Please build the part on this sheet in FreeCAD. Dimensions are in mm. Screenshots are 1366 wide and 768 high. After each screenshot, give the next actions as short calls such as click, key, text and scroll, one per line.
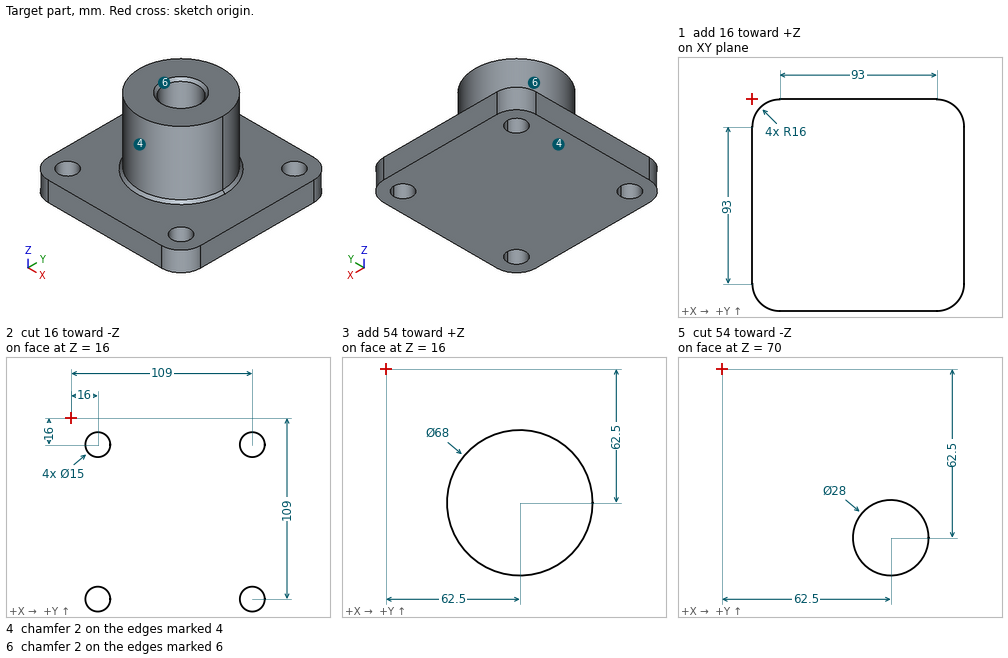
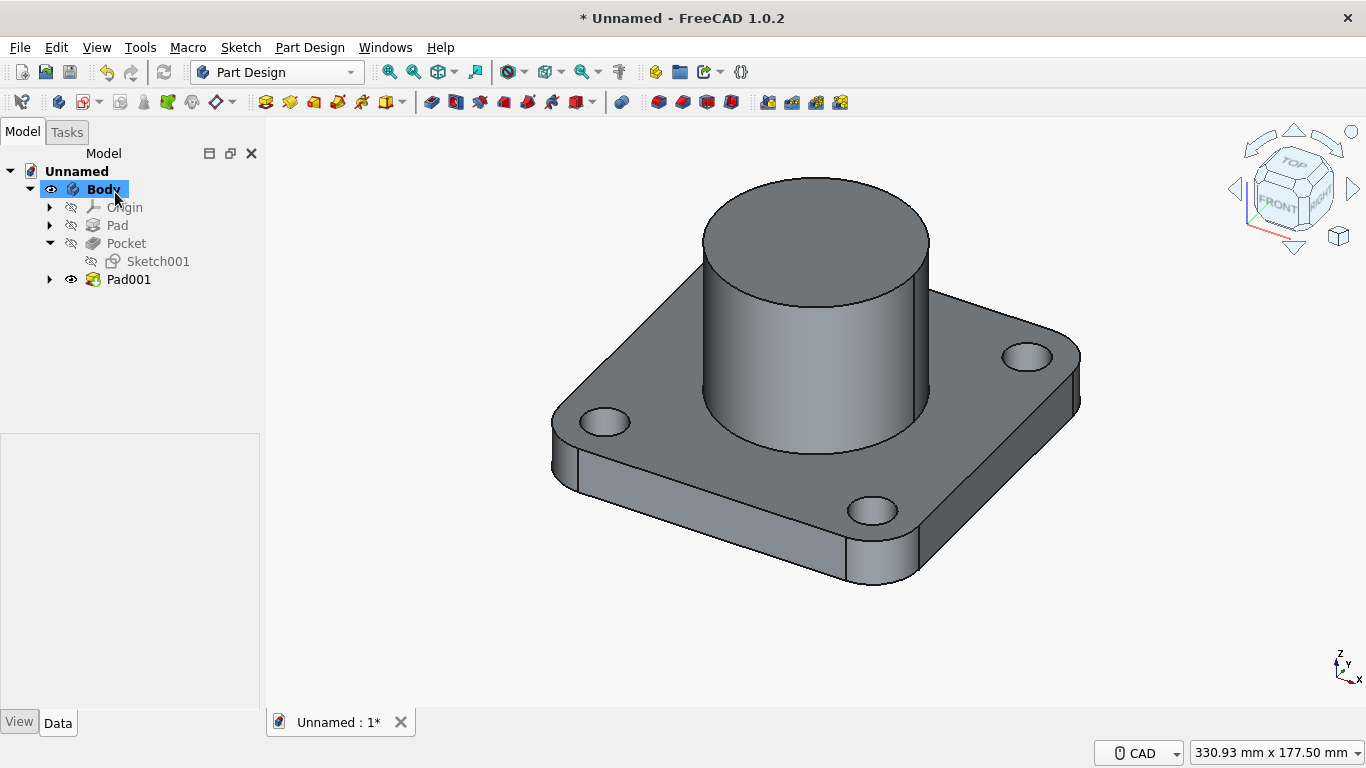
key(v)
key(f)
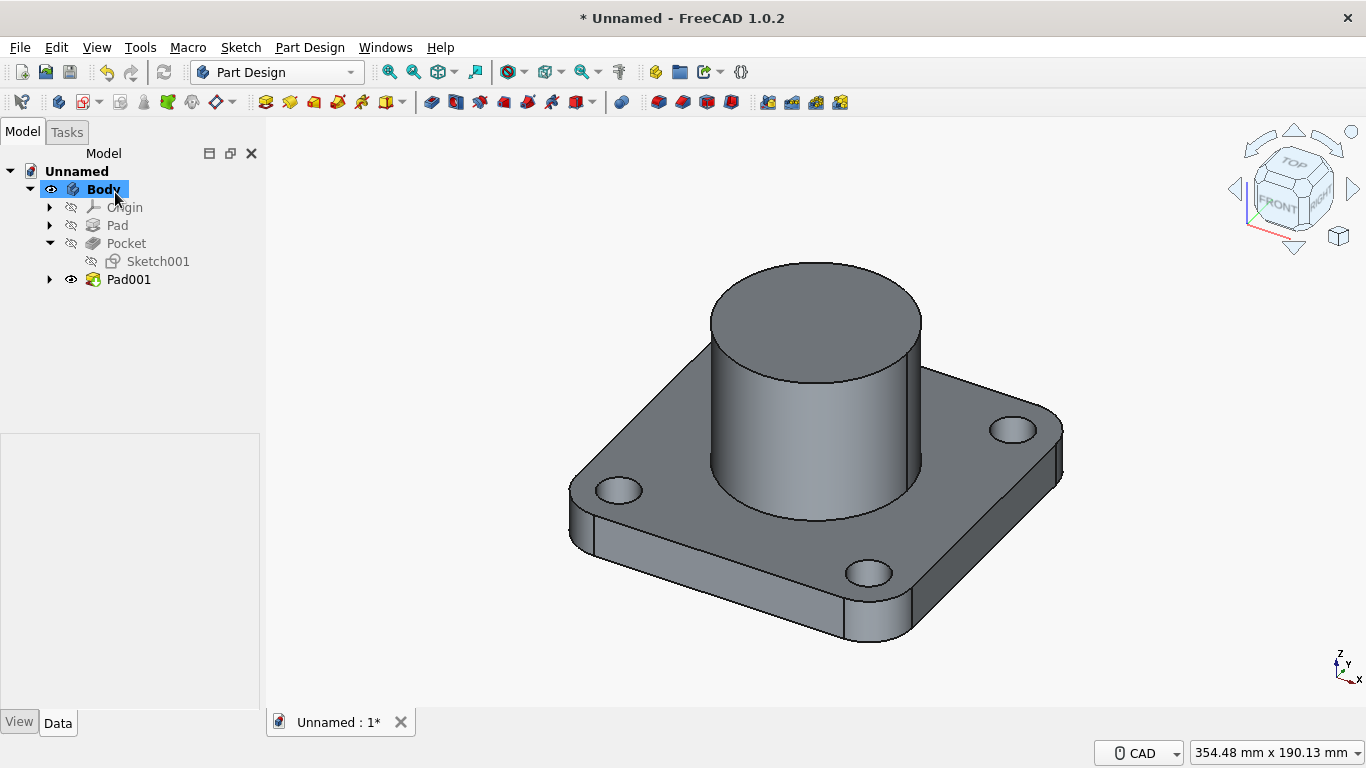
key(0)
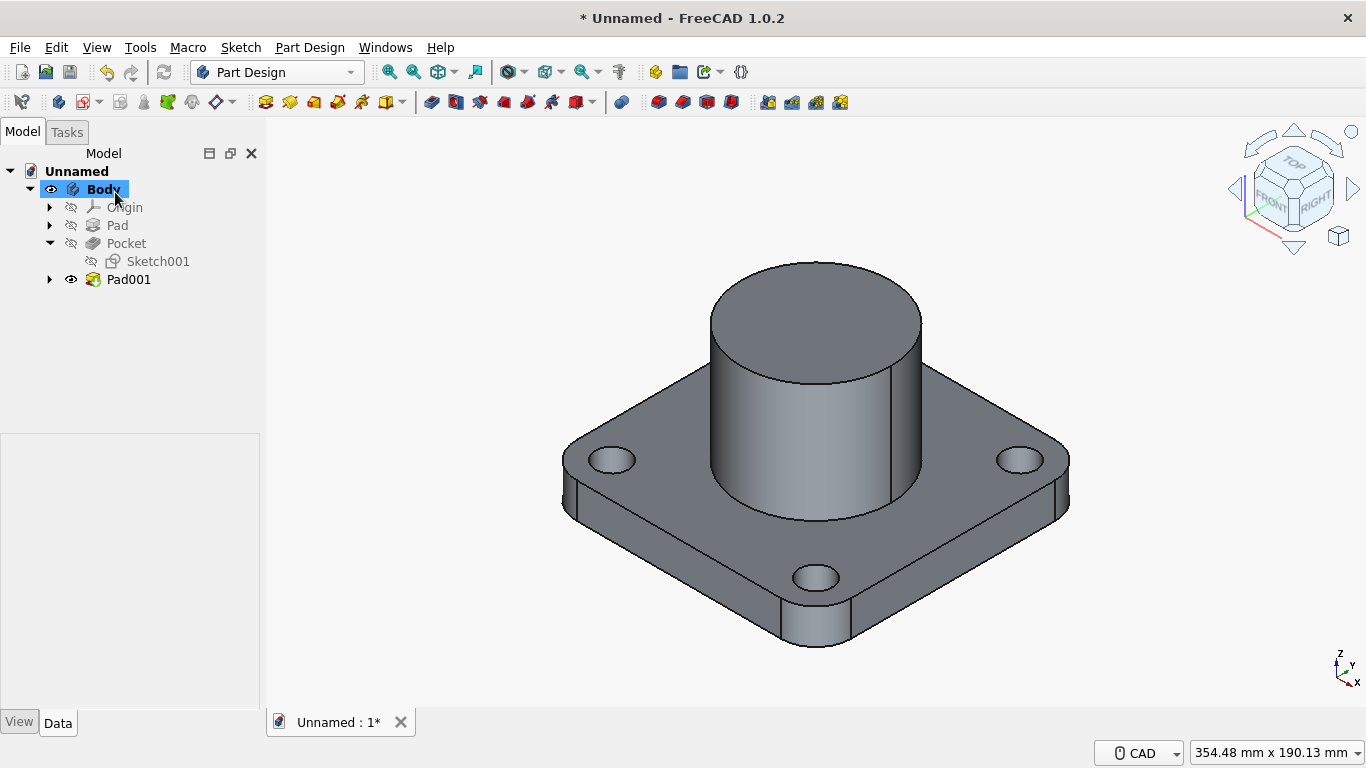
key(2)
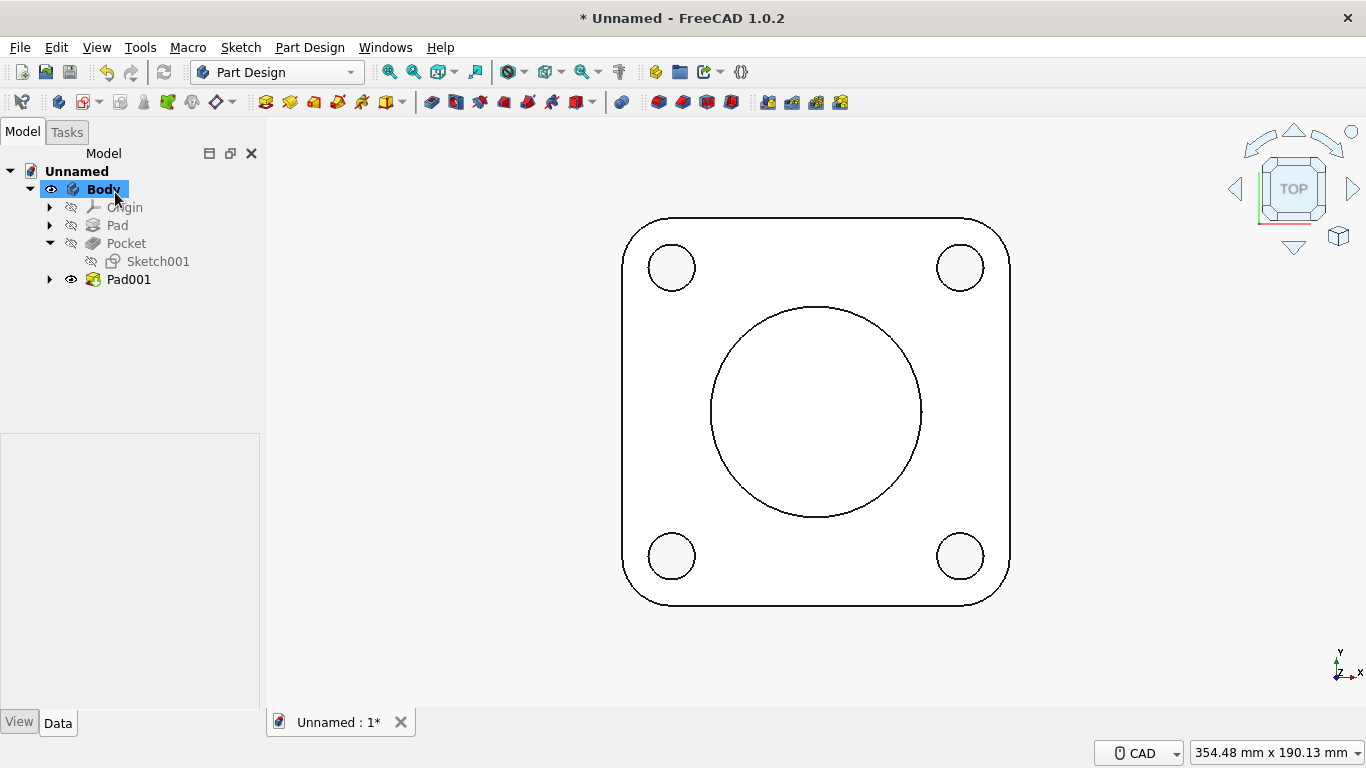
key(1)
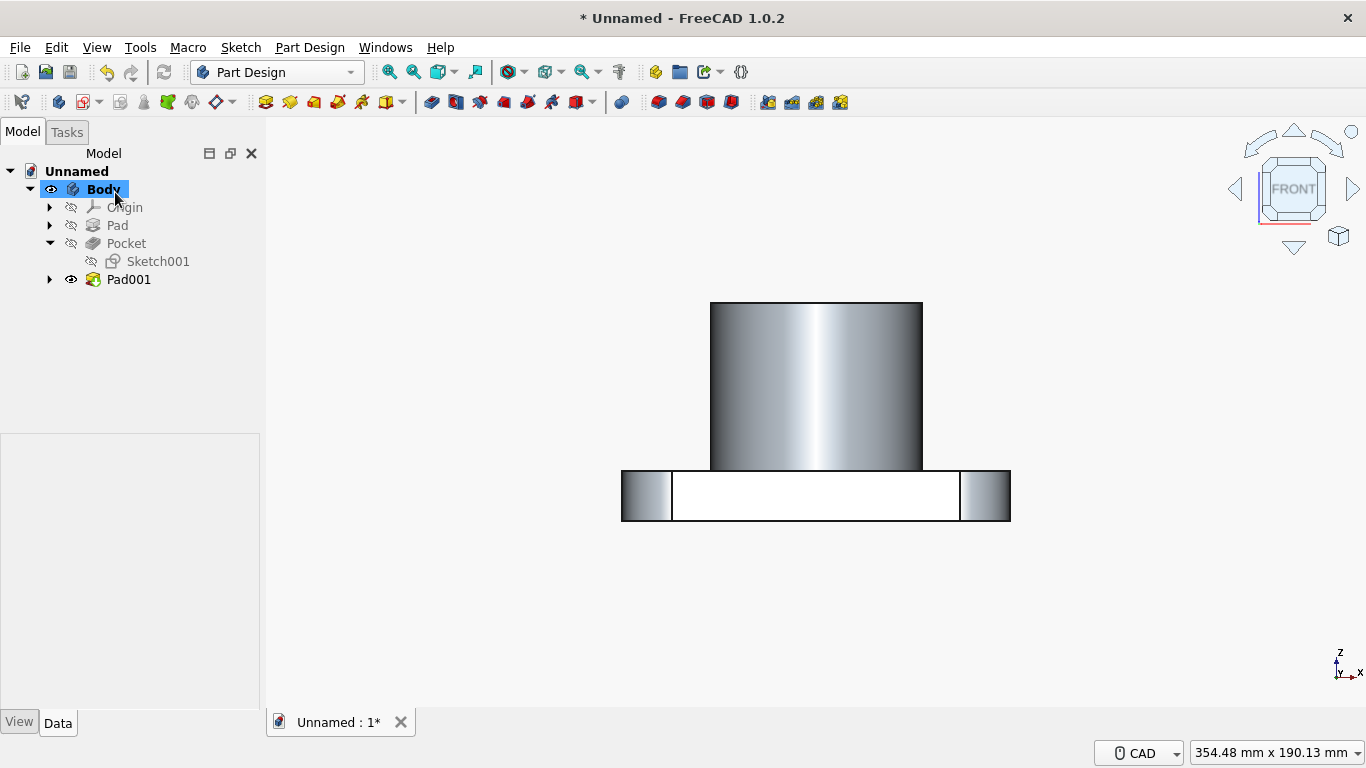
key(v)
key(f)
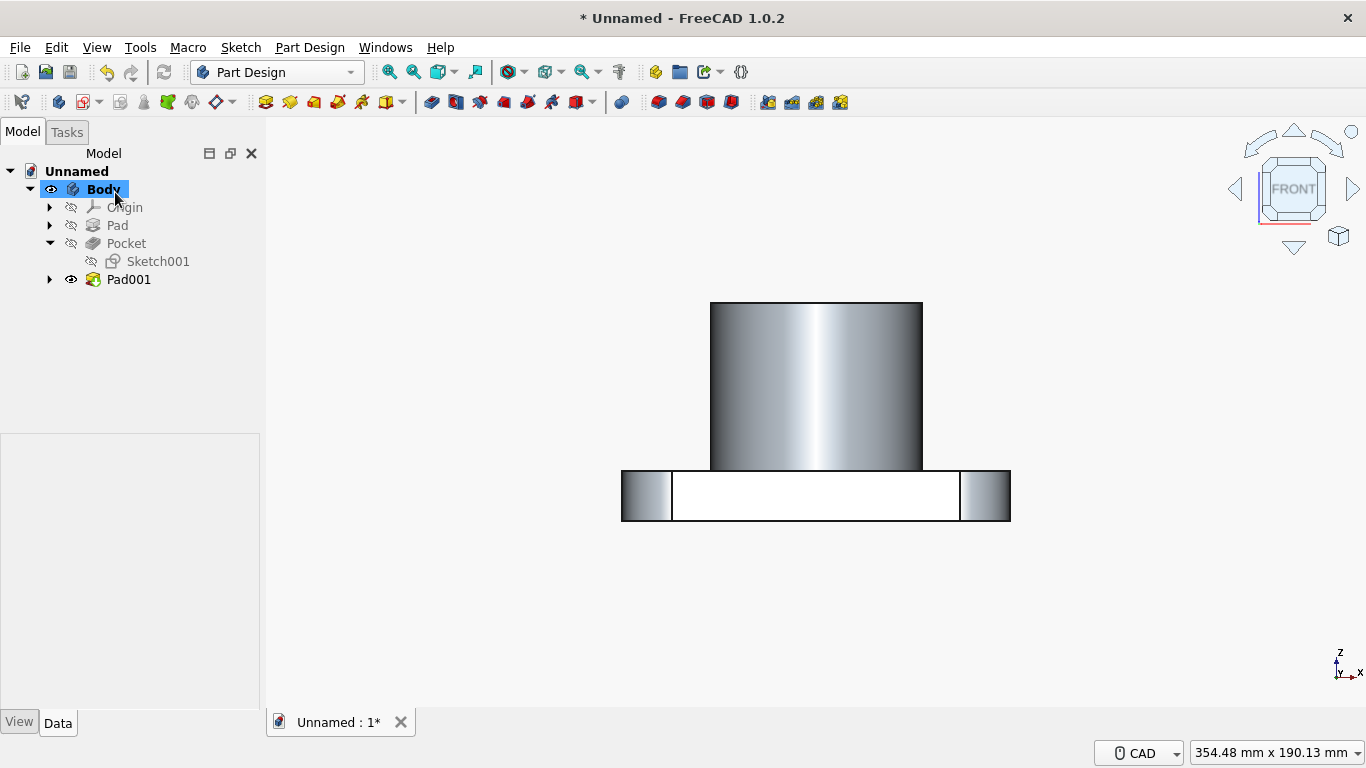
key(3)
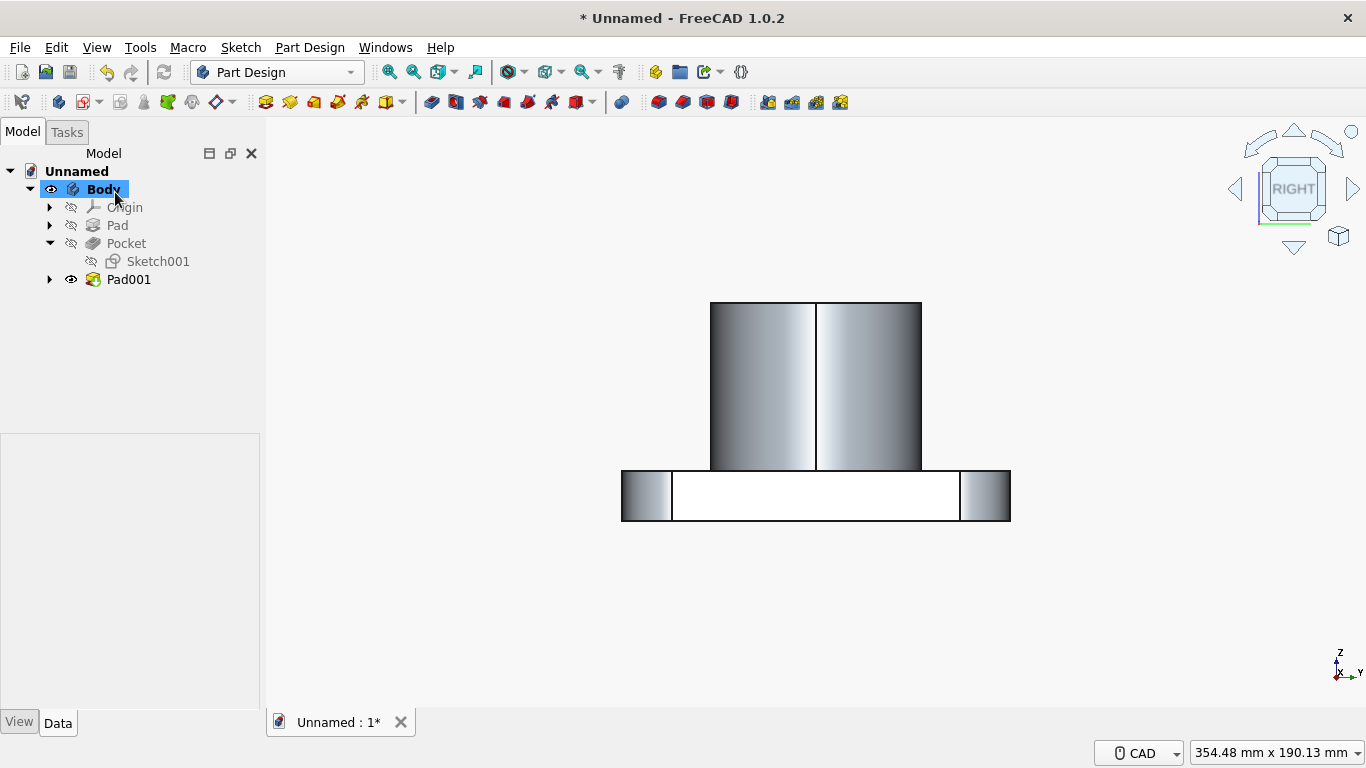
key(v)
key(f)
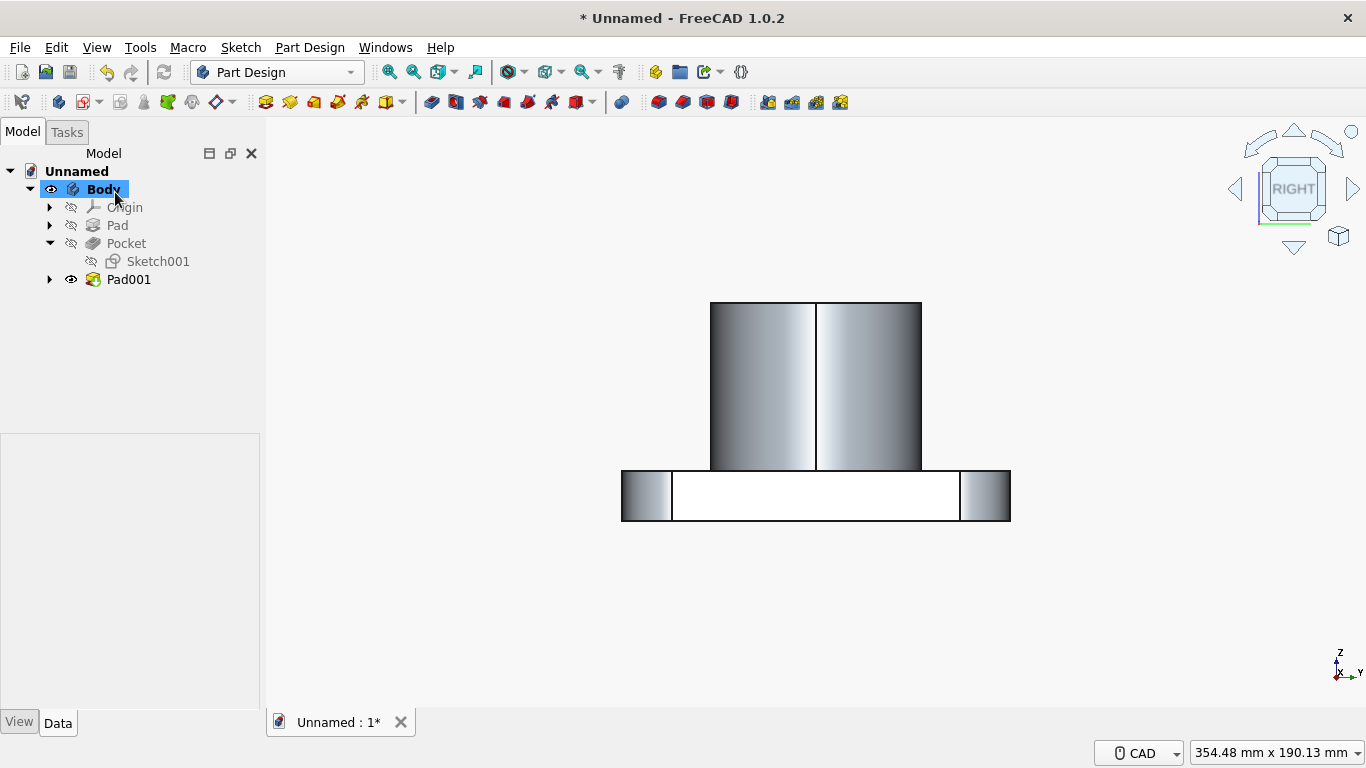
key(5)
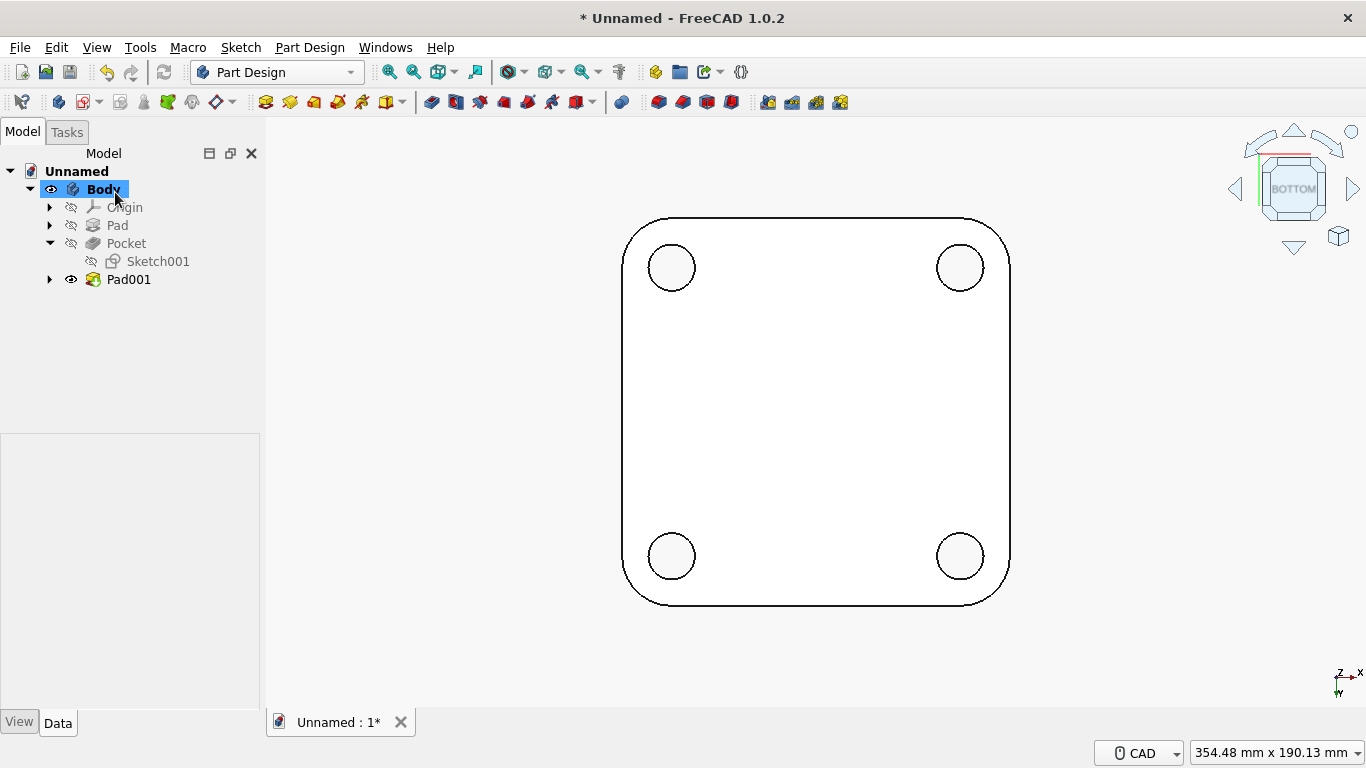
key(4)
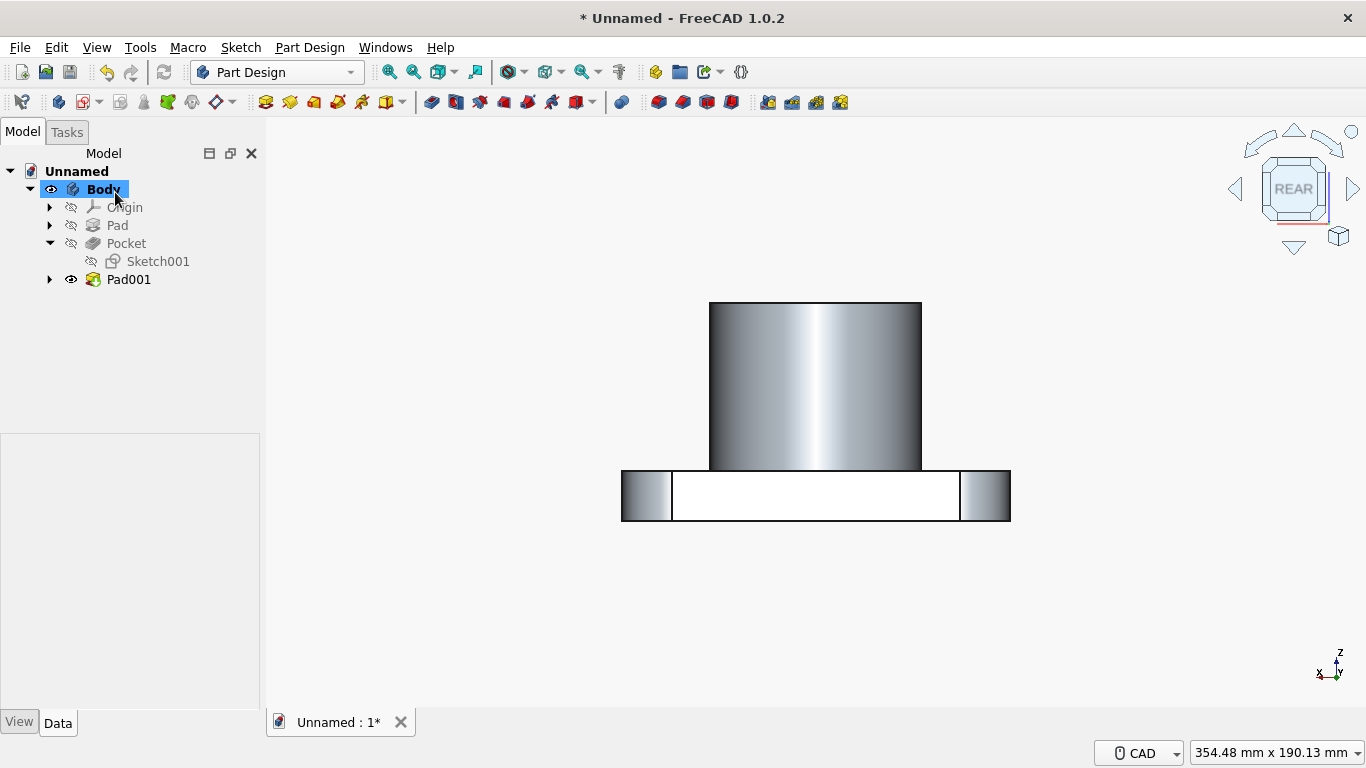
key(v)
key(f)